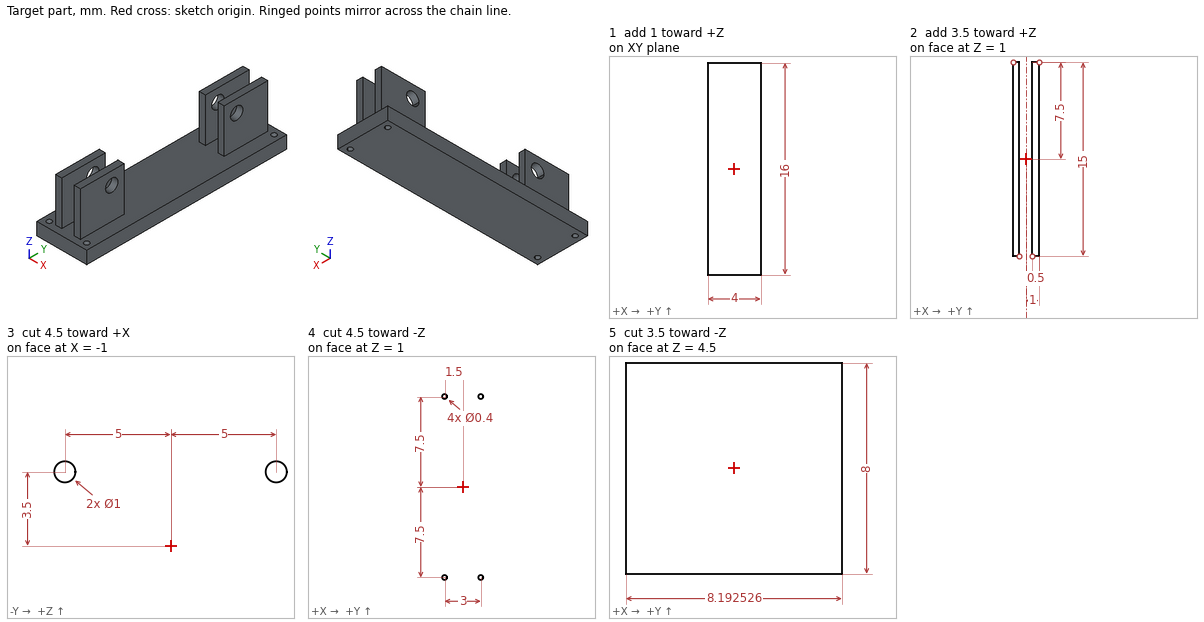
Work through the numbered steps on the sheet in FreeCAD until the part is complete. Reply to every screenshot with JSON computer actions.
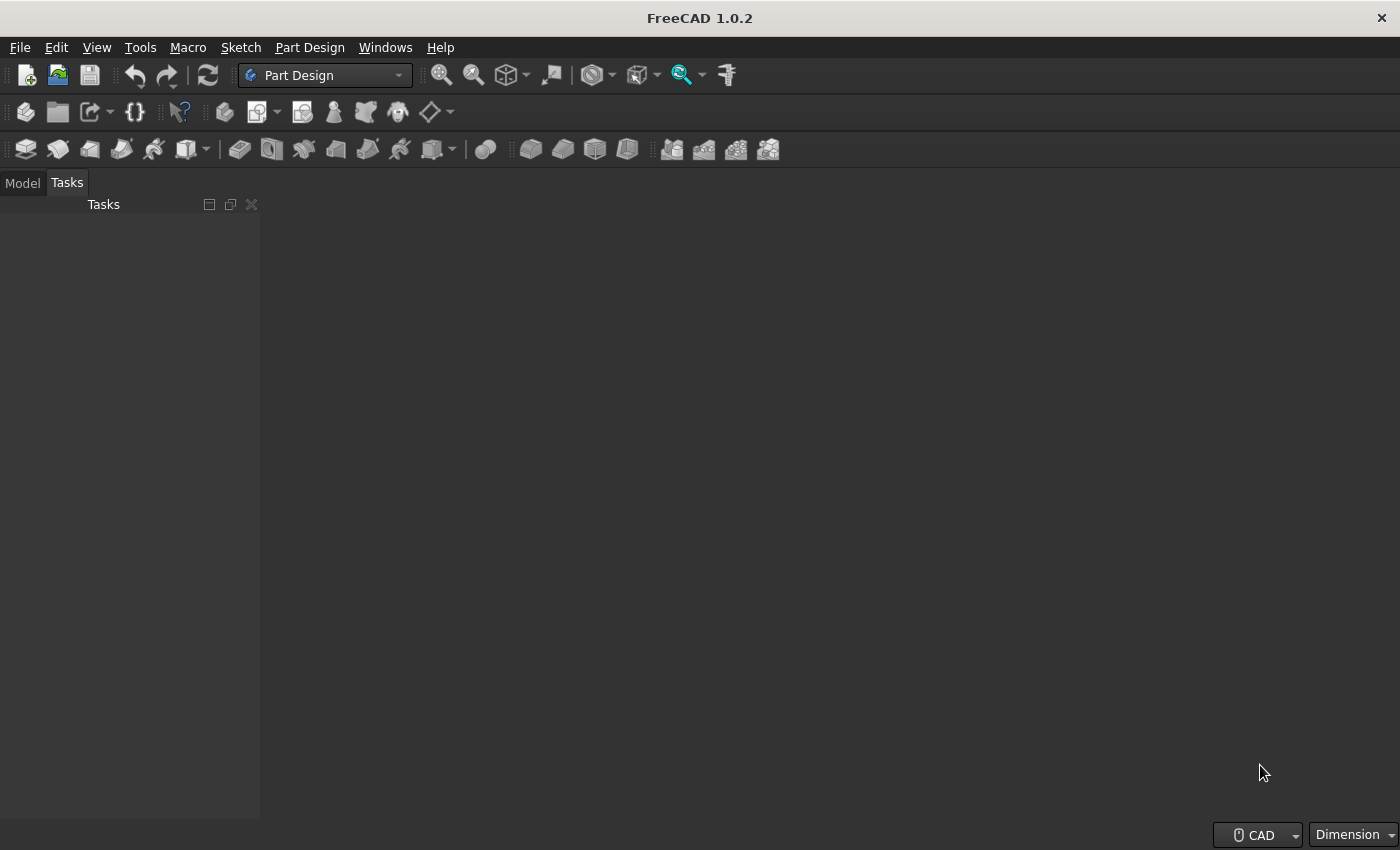
{"action": "key", "text": "ctrl+n"}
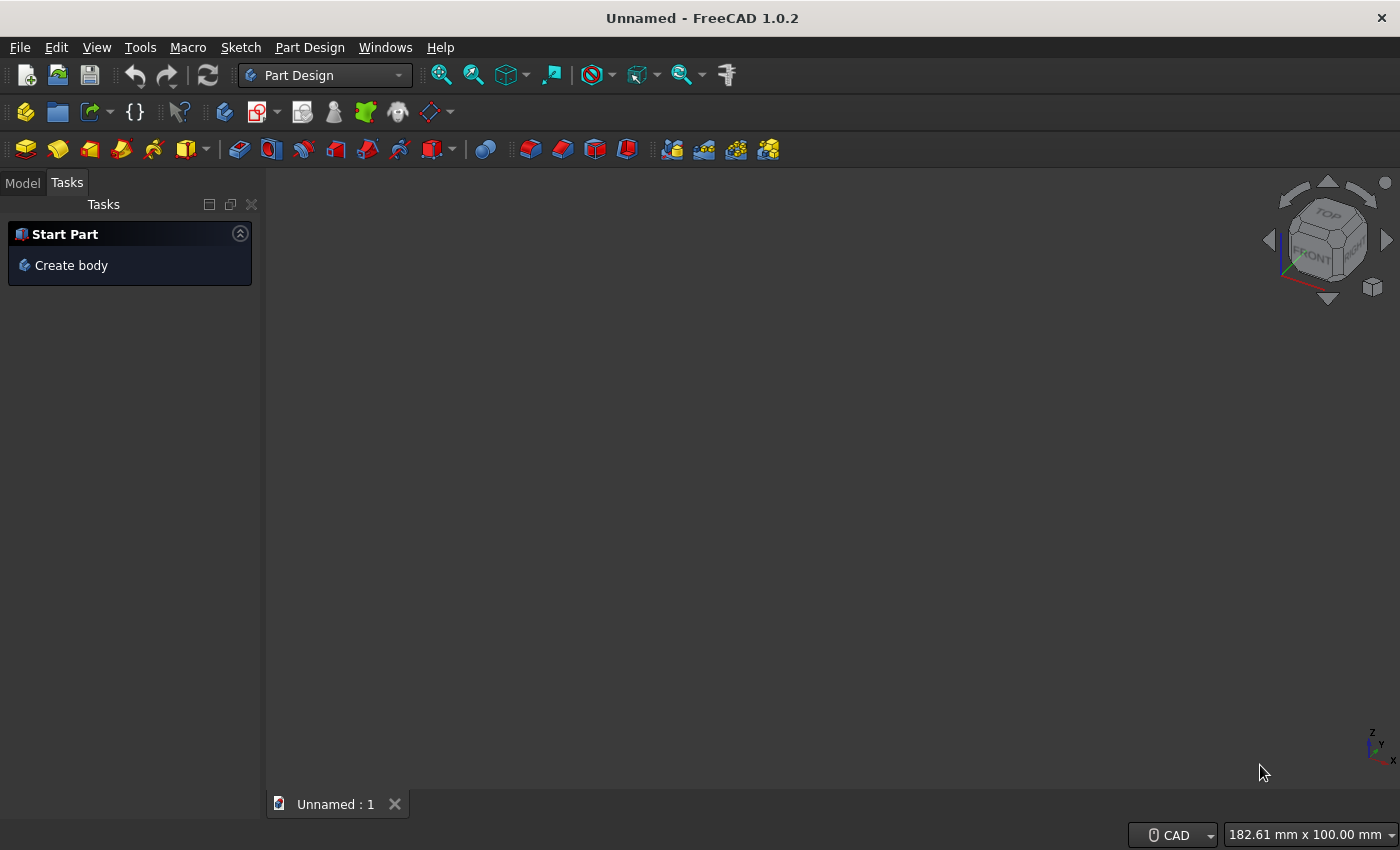
{"action": "left_click", "coordinate": [258, 112]}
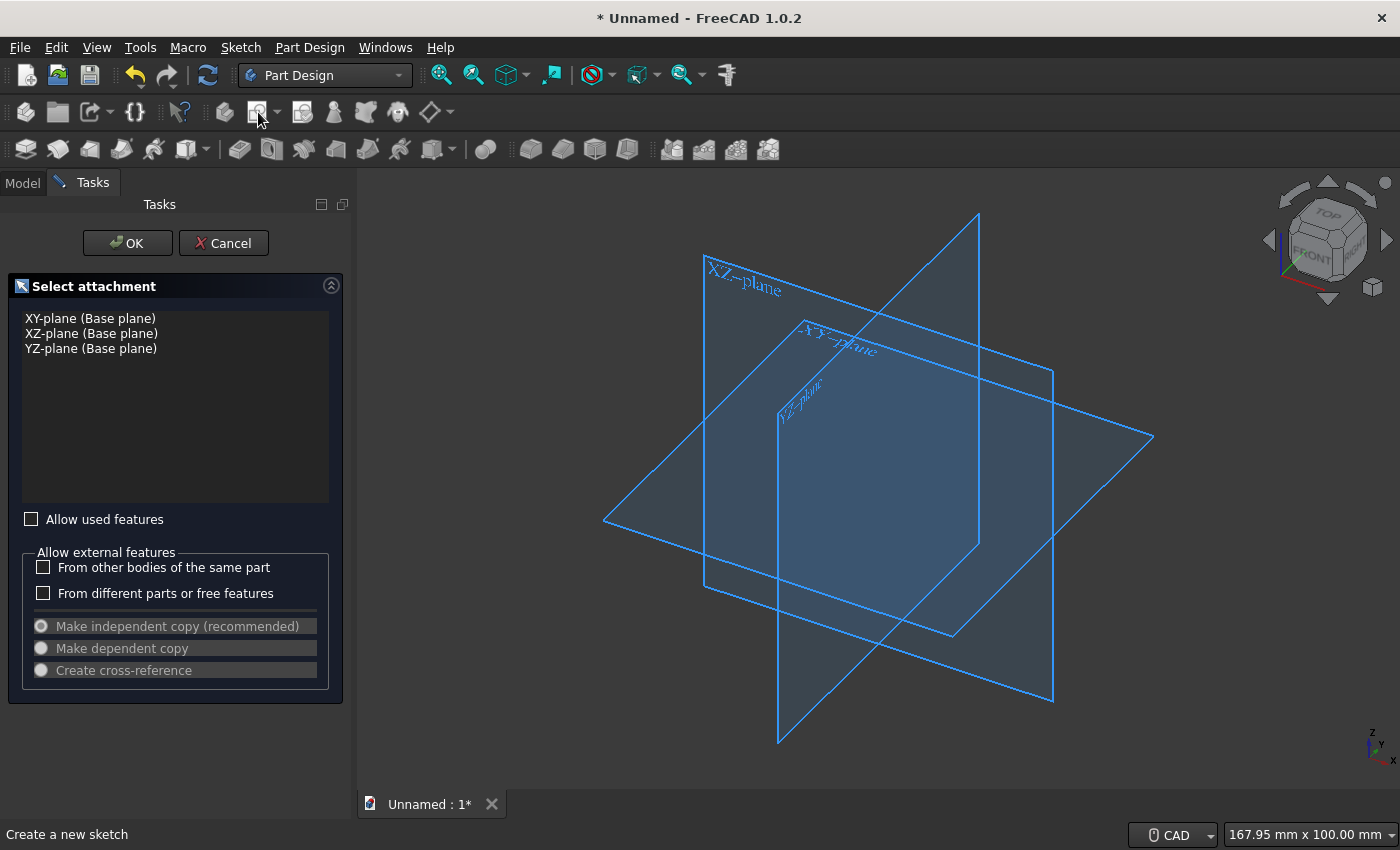
{"action": "left_click", "coordinate": [82, 318]}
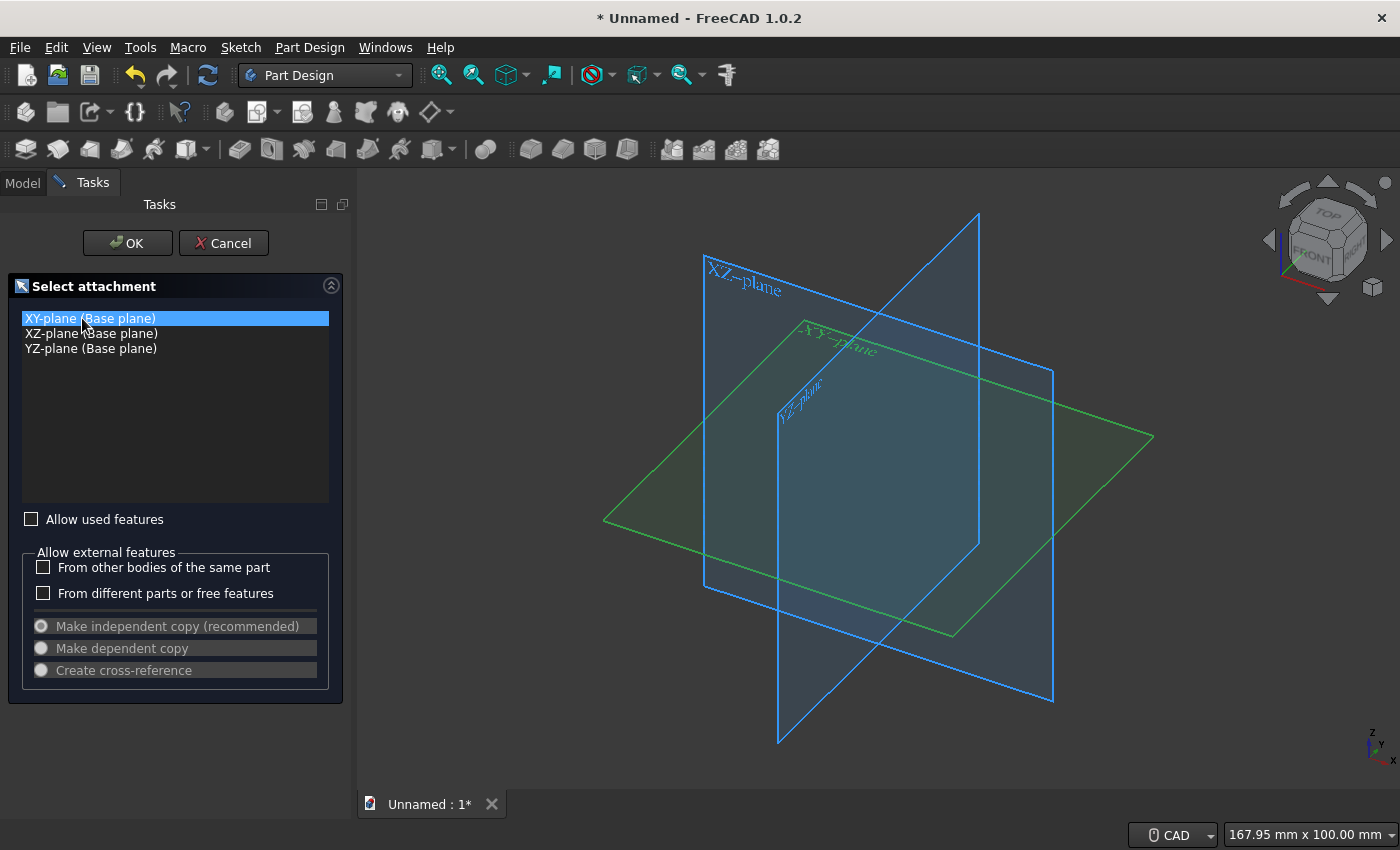
{"action": "left_click", "coordinate": [128, 243]}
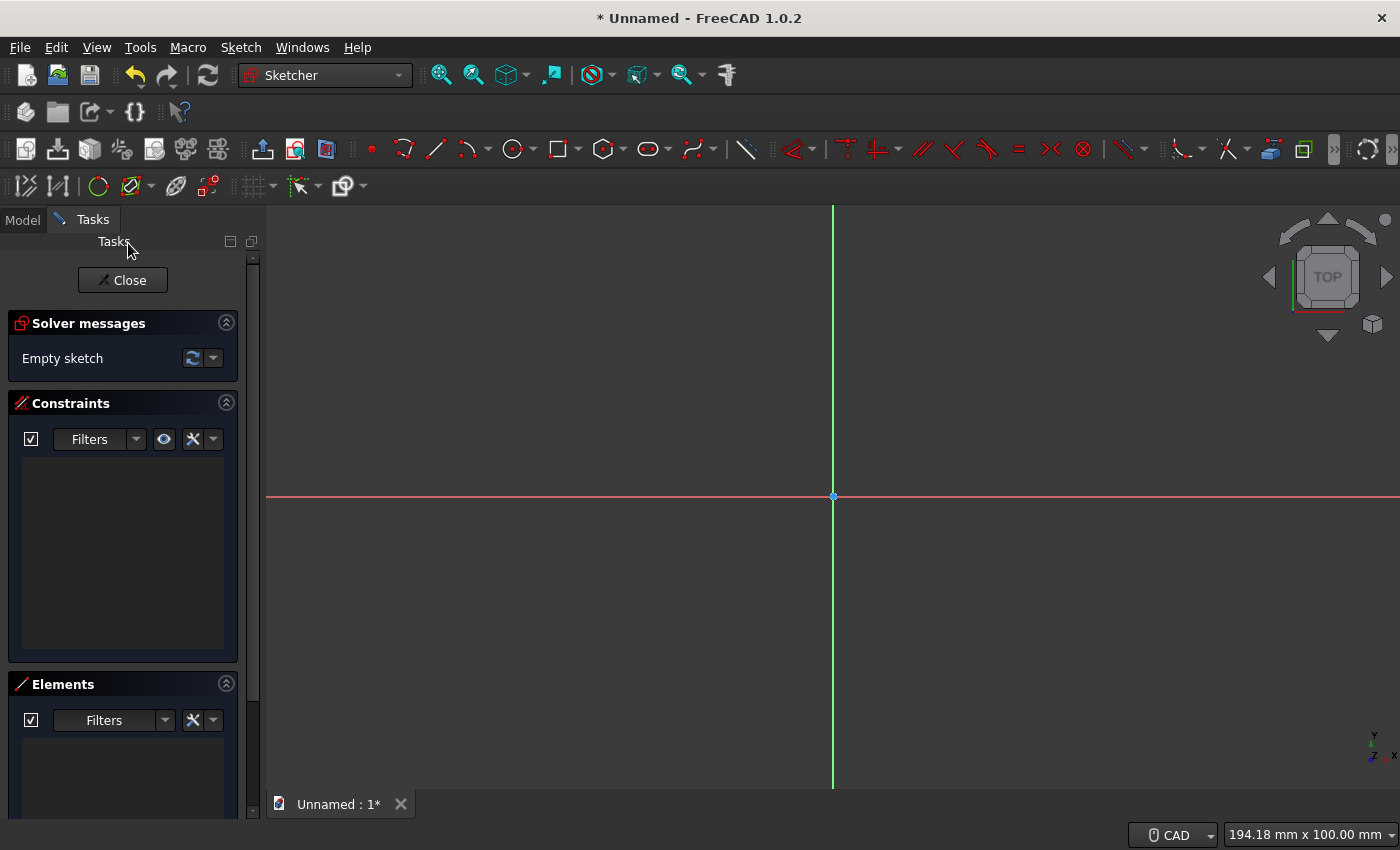
{"action": "scroll", "coordinate": [855, 497], "scroll_direction": "up", "scroll_amount": 7}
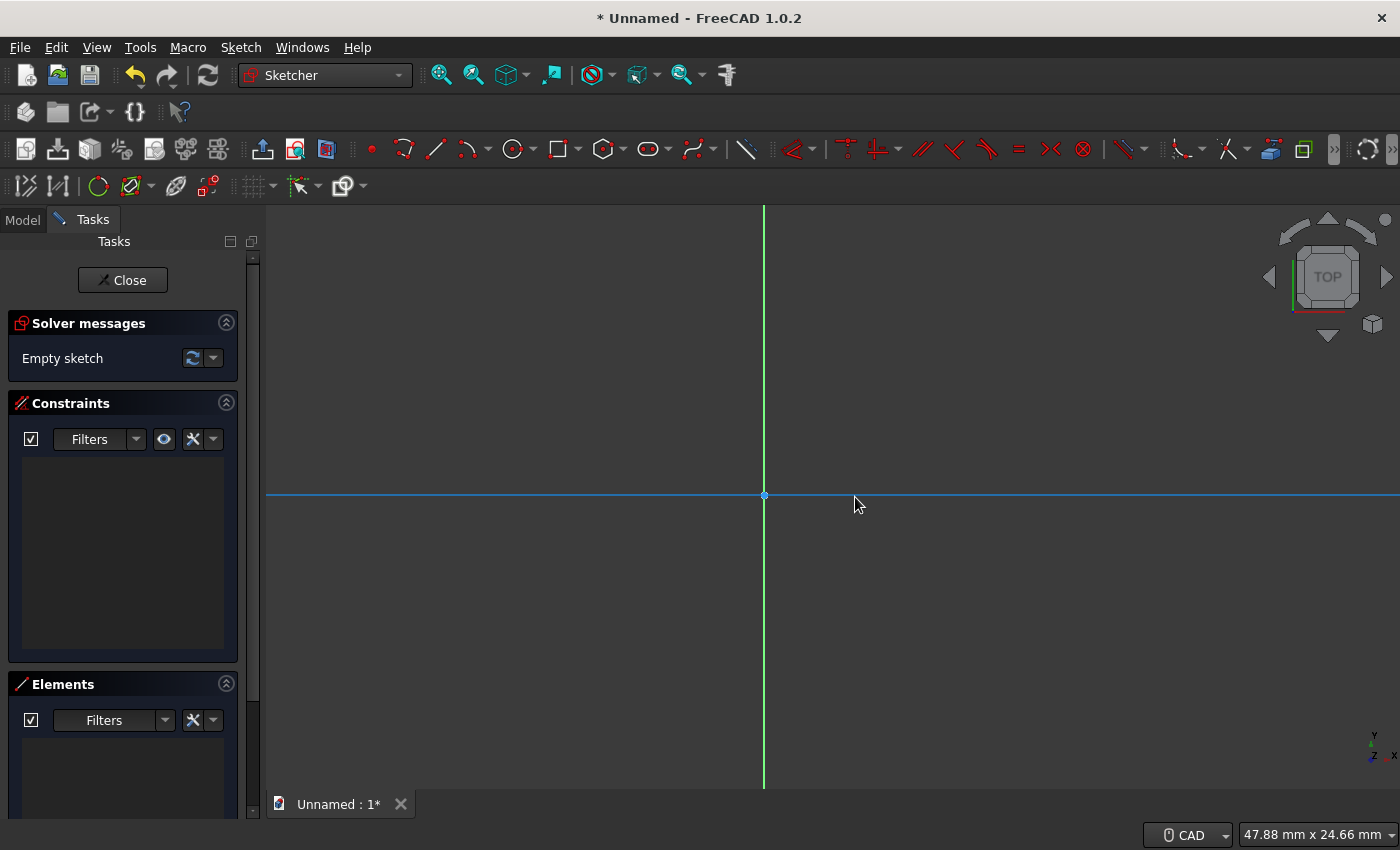
{"action": "key", "text": "g v"}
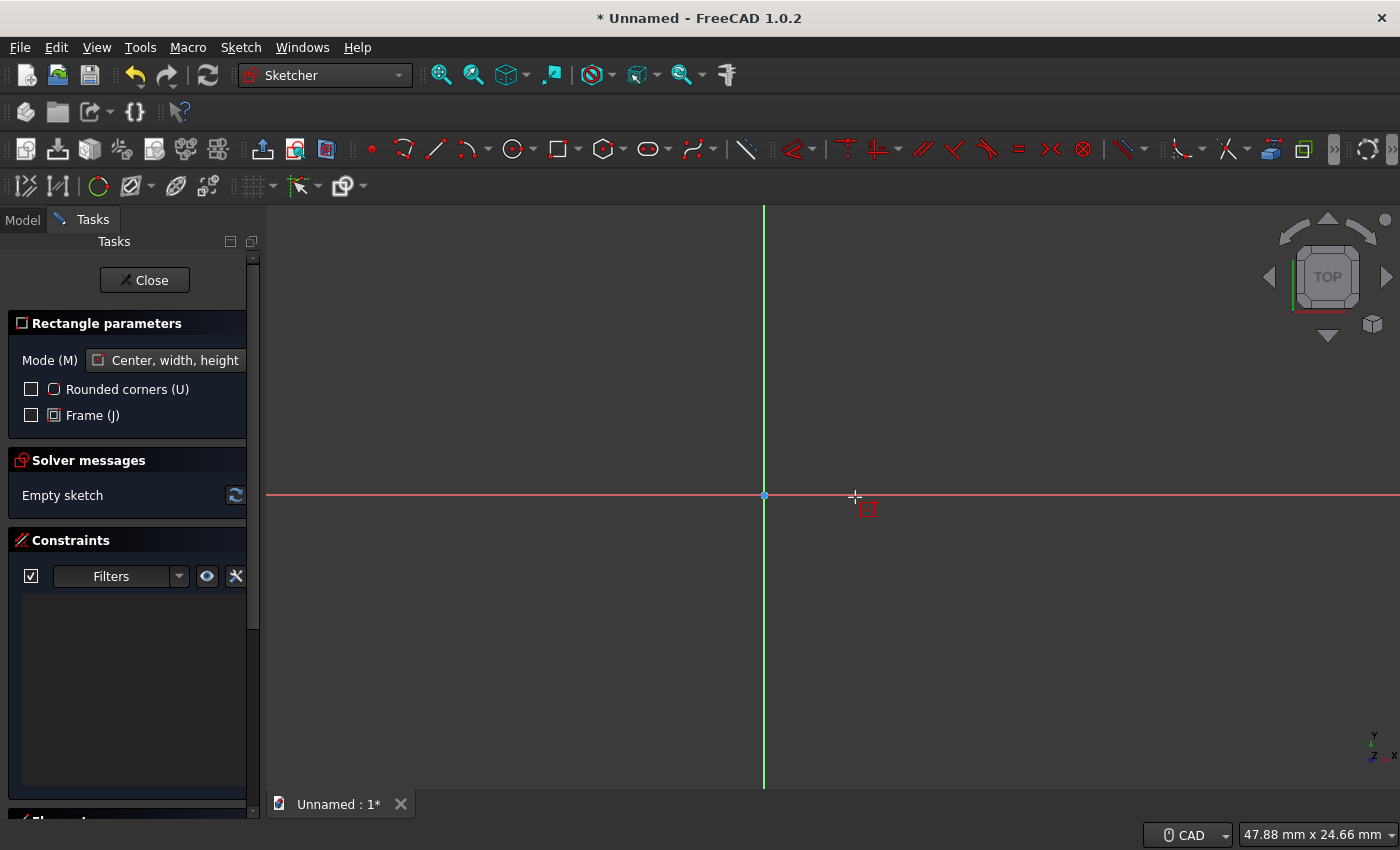
{"action": "left_click", "coordinate": [764, 495]}
{"action": "left_click", "coordinate": [812, 306]}
{"action": "key", "text": "Escape"}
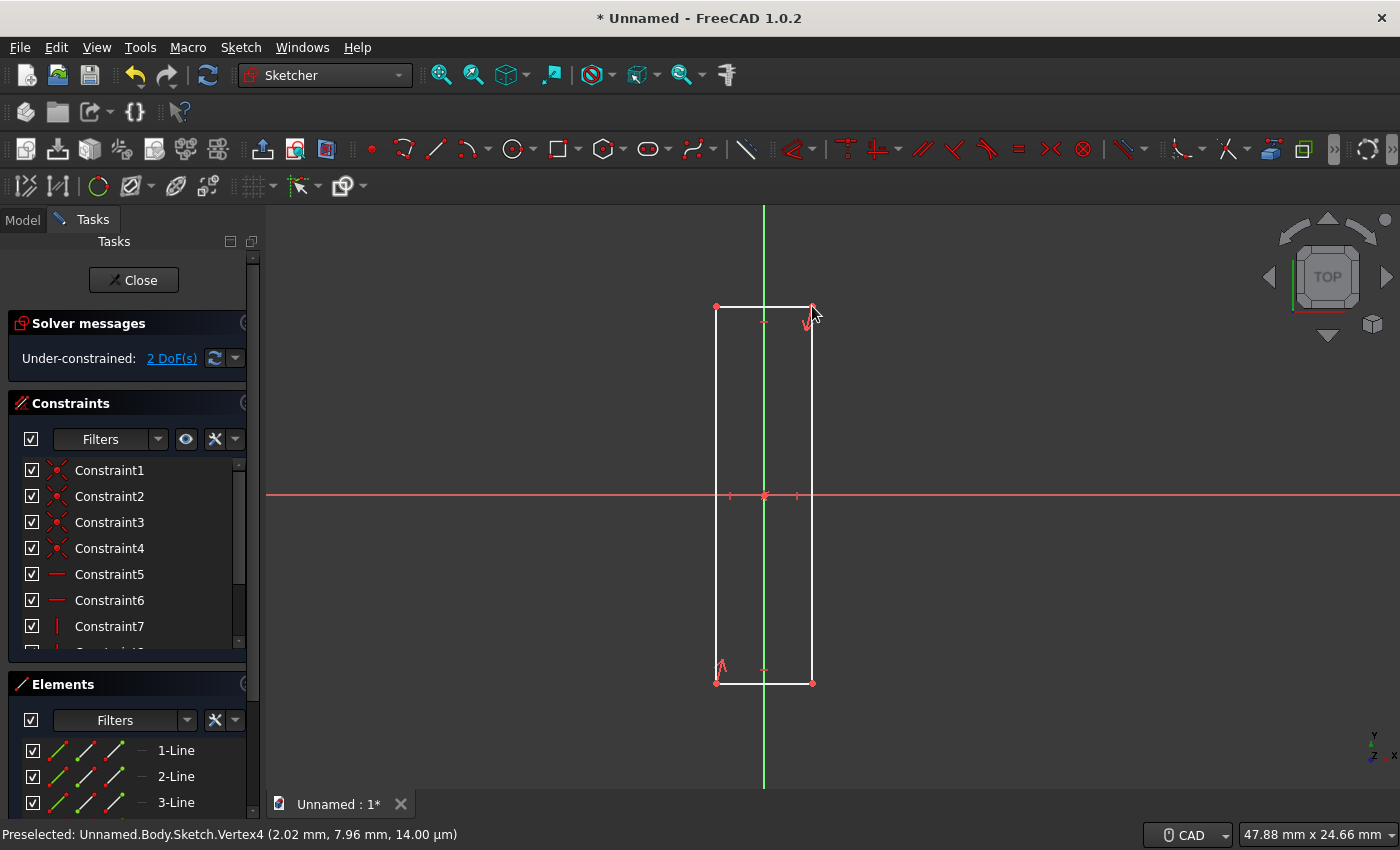
{"action": "left_click", "coordinate": [792, 150]}